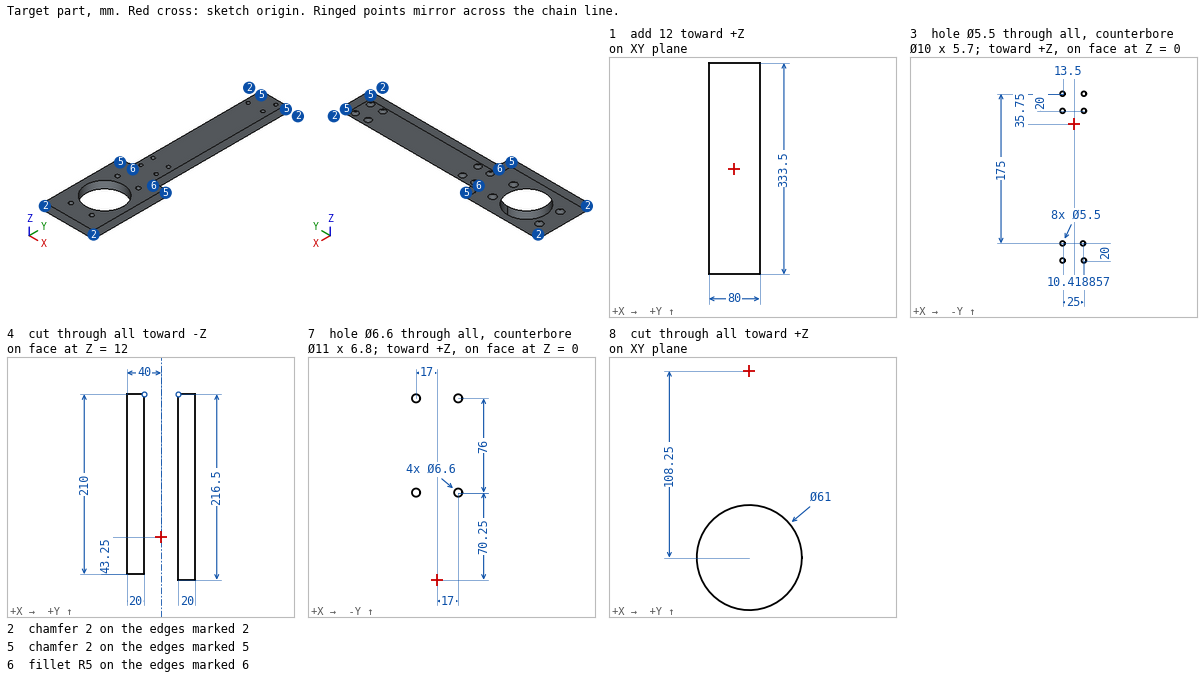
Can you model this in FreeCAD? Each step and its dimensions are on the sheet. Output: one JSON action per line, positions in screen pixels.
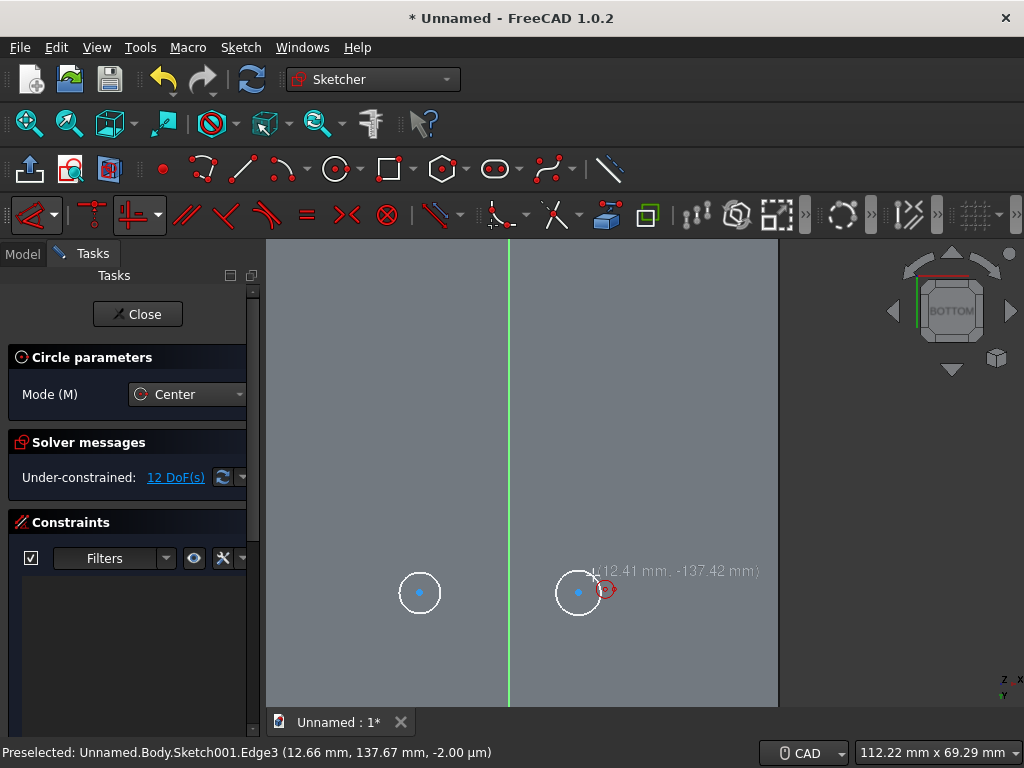
{"action": "scroll", "coordinate": [595, 576], "scroll_direction": "down", "scroll_amount": 8}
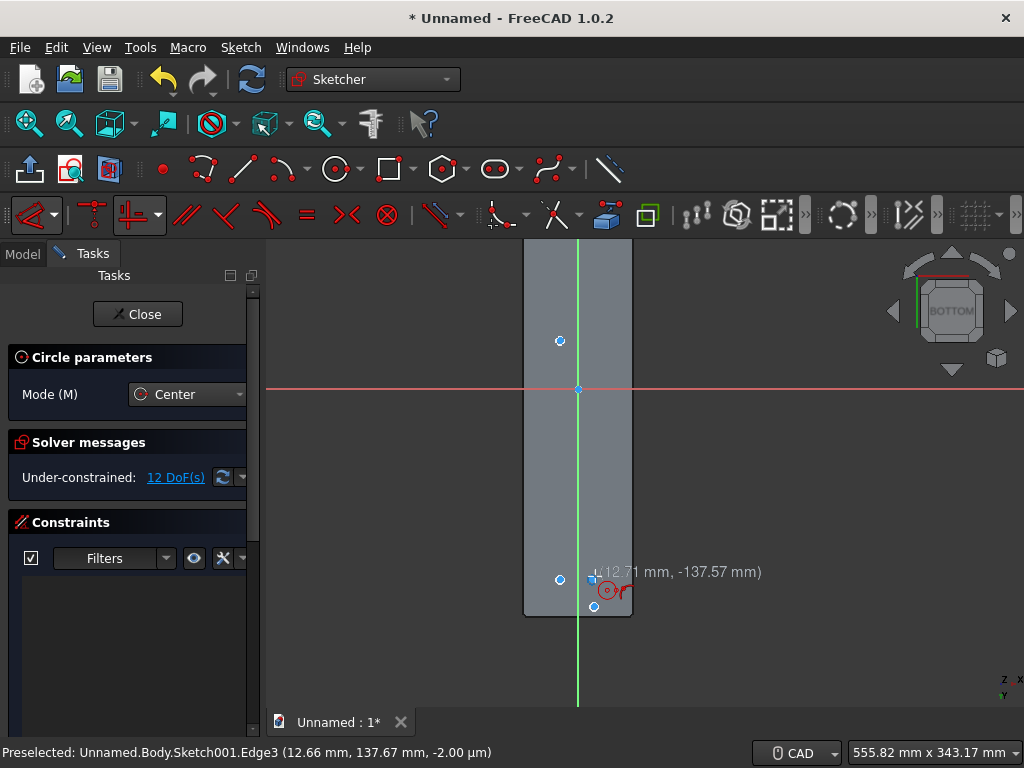
{"action": "scroll", "coordinate": [560, 606], "scroll_direction": "up", "scroll_amount": 9}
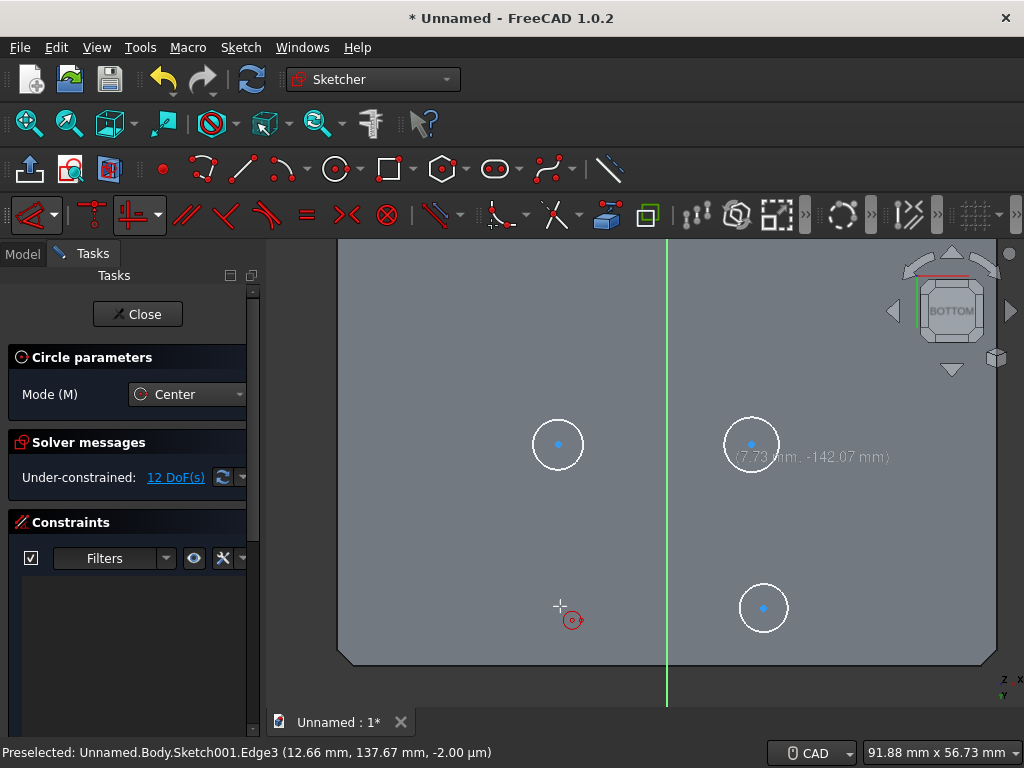
{"action": "scroll", "coordinate": [560, 606], "scroll_direction": "down", "scroll_amount": 9}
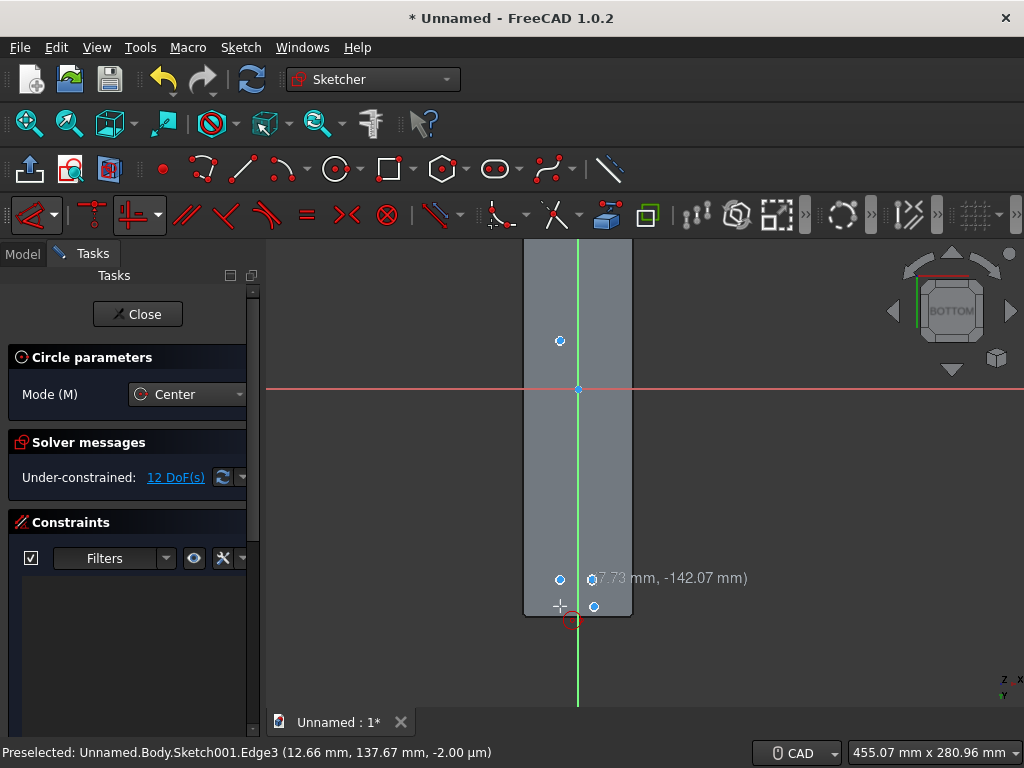
{"action": "left_click", "coordinate": [560, 606]}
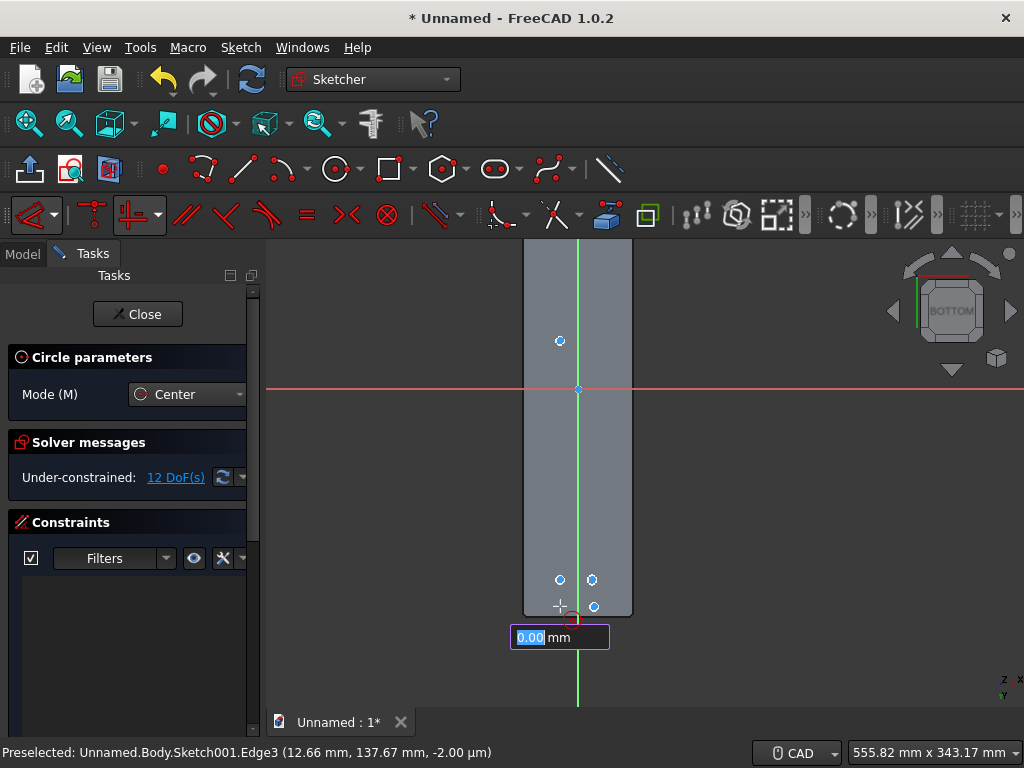
{"action": "scroll", "coordinate": [562, 604], "scroll_direction": "up", "scroll_amount": 8}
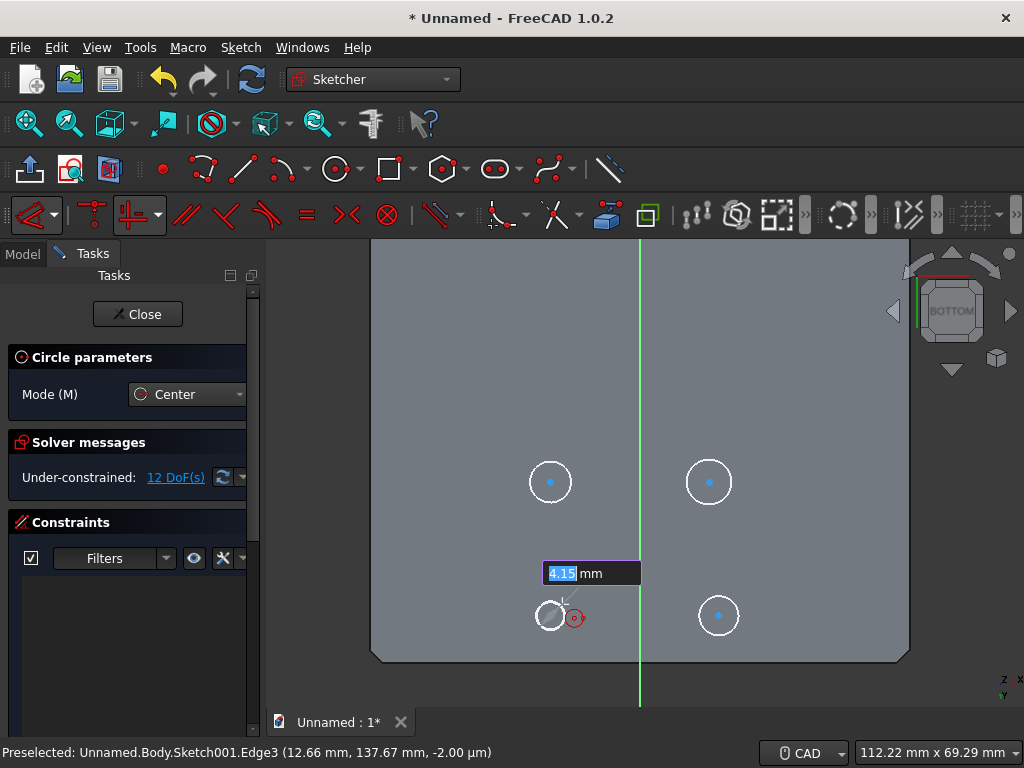
{"action": "left_click", "coordinate": [562, 599]}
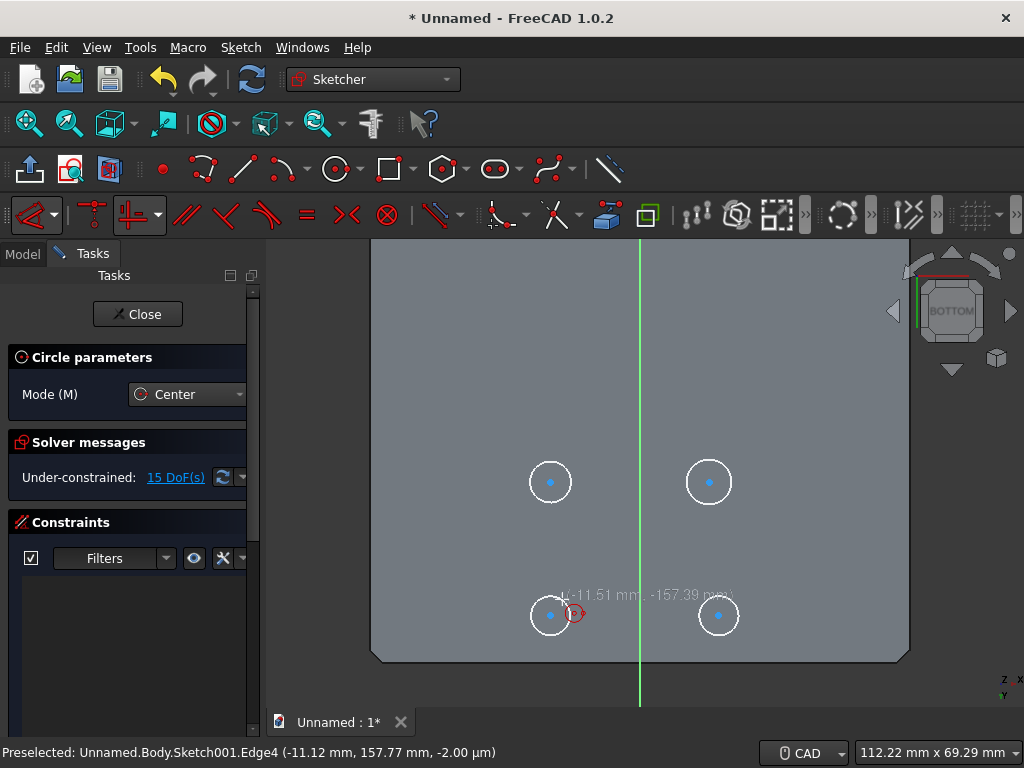
{"action": "scroll", "coordinate": [562, 604], "scroll_direction": "down", "scroll_amount": 8}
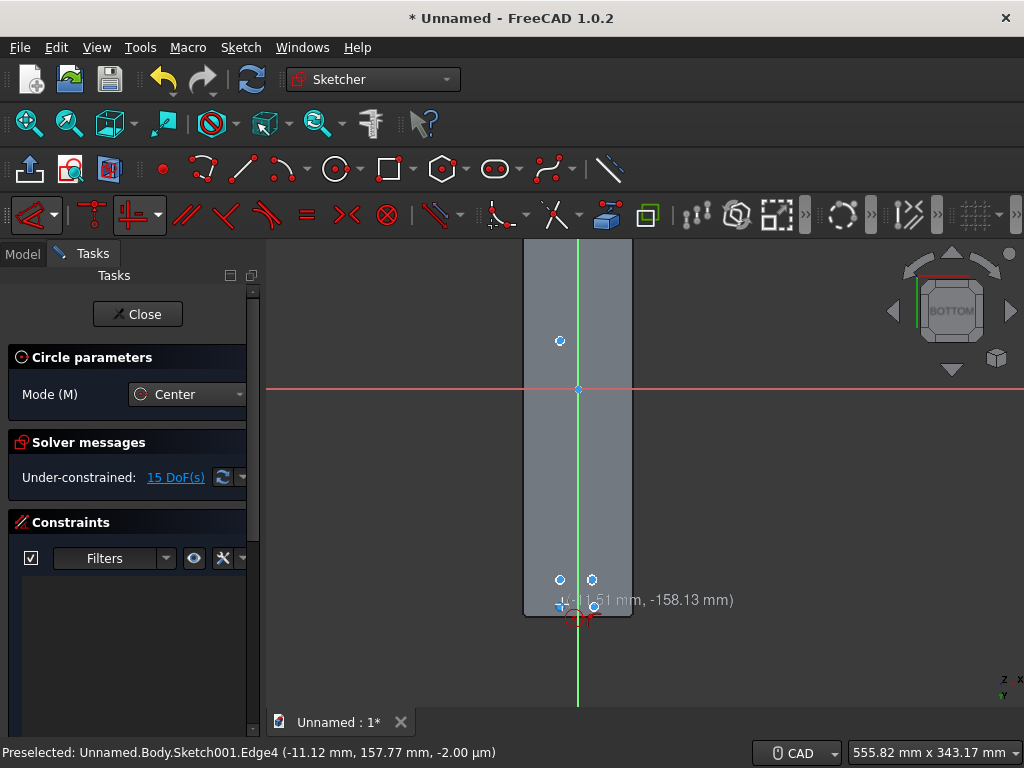
{"action": "scroll", "coordinate": [594, 368], "scroll_direction": "up", "scroll_amount": 9}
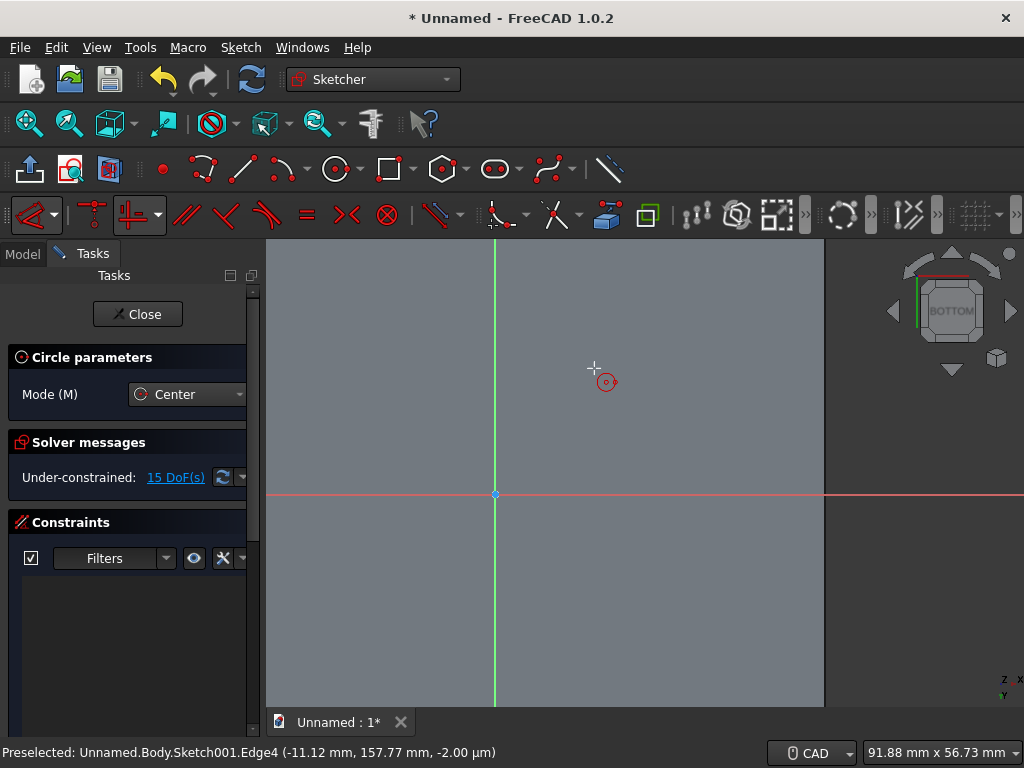
{"action": "scroll", "coordinate": [594, 368], "scroll_direction": "down", "scroll_amount": 9}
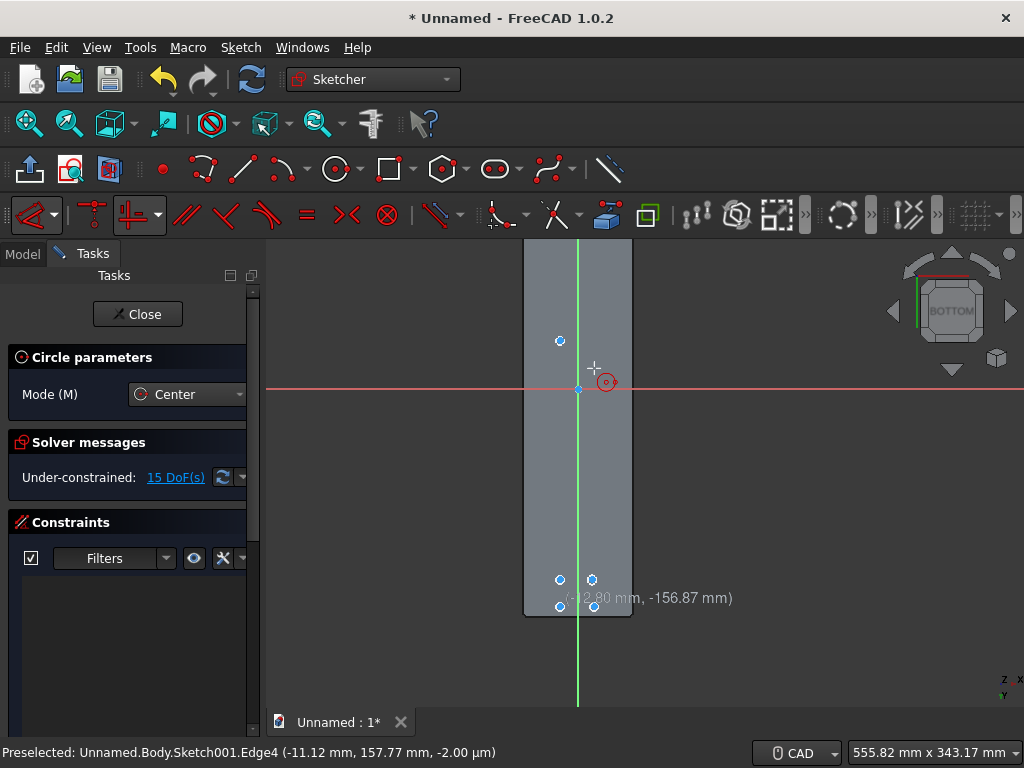
{"action": "left_click", "coordinate": [594, 368]}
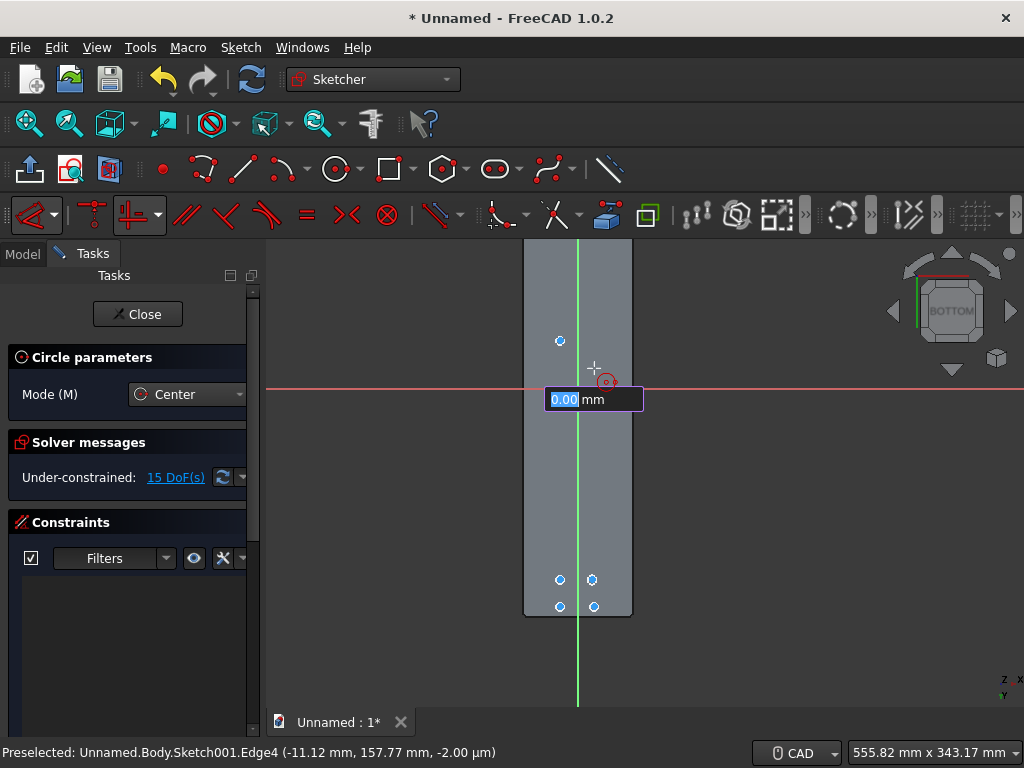
{"action": "scroll", "coordinate": [596, 365], "scroll_direction": "up", "scroll_amount": 8}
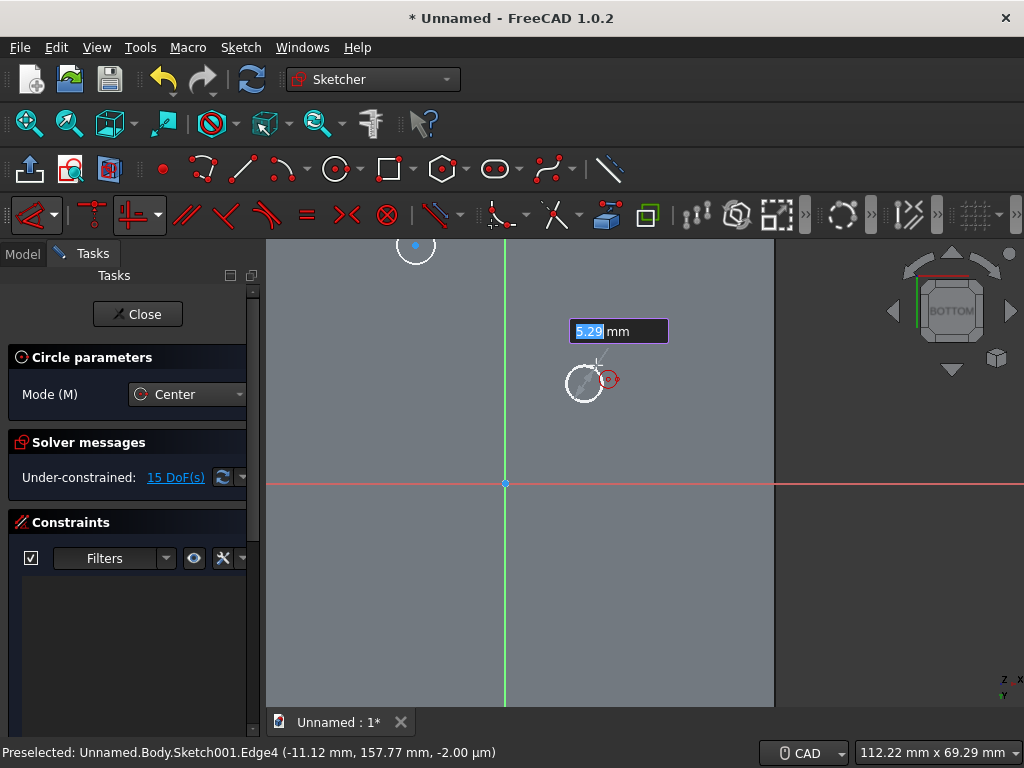
{"action": "left_click", "coordinate": [596, 364]}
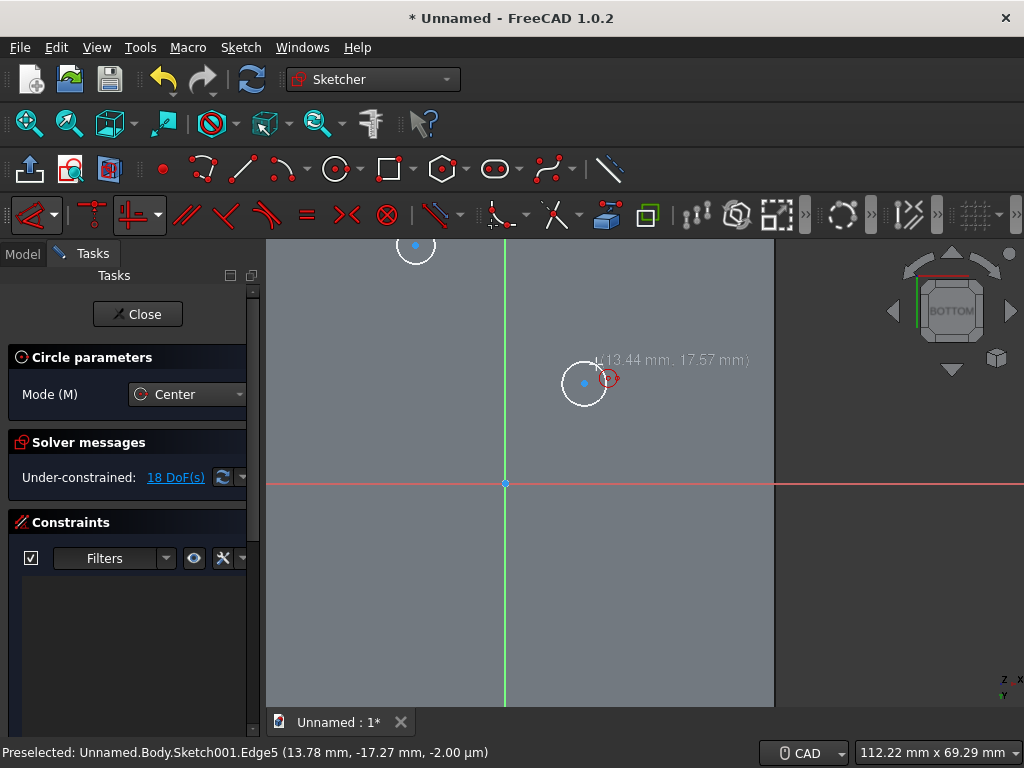
{"action": "scroll", "coordinate": [596, 365], "scroll_direction": "down", "scroll_amount": 8}